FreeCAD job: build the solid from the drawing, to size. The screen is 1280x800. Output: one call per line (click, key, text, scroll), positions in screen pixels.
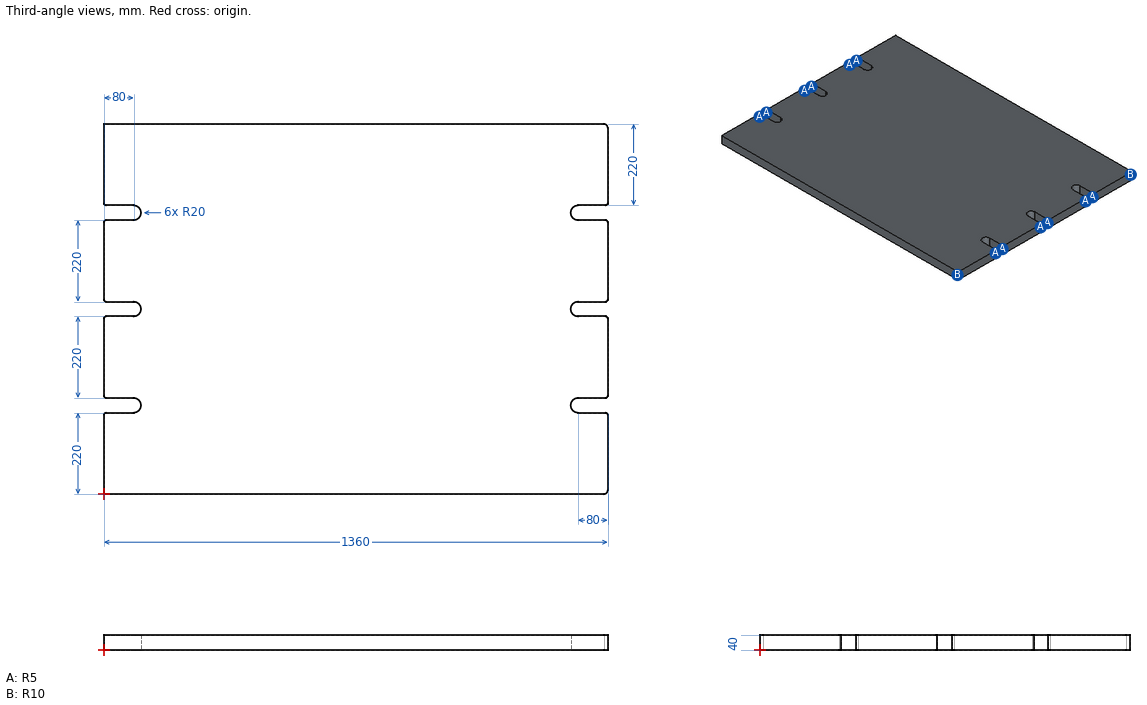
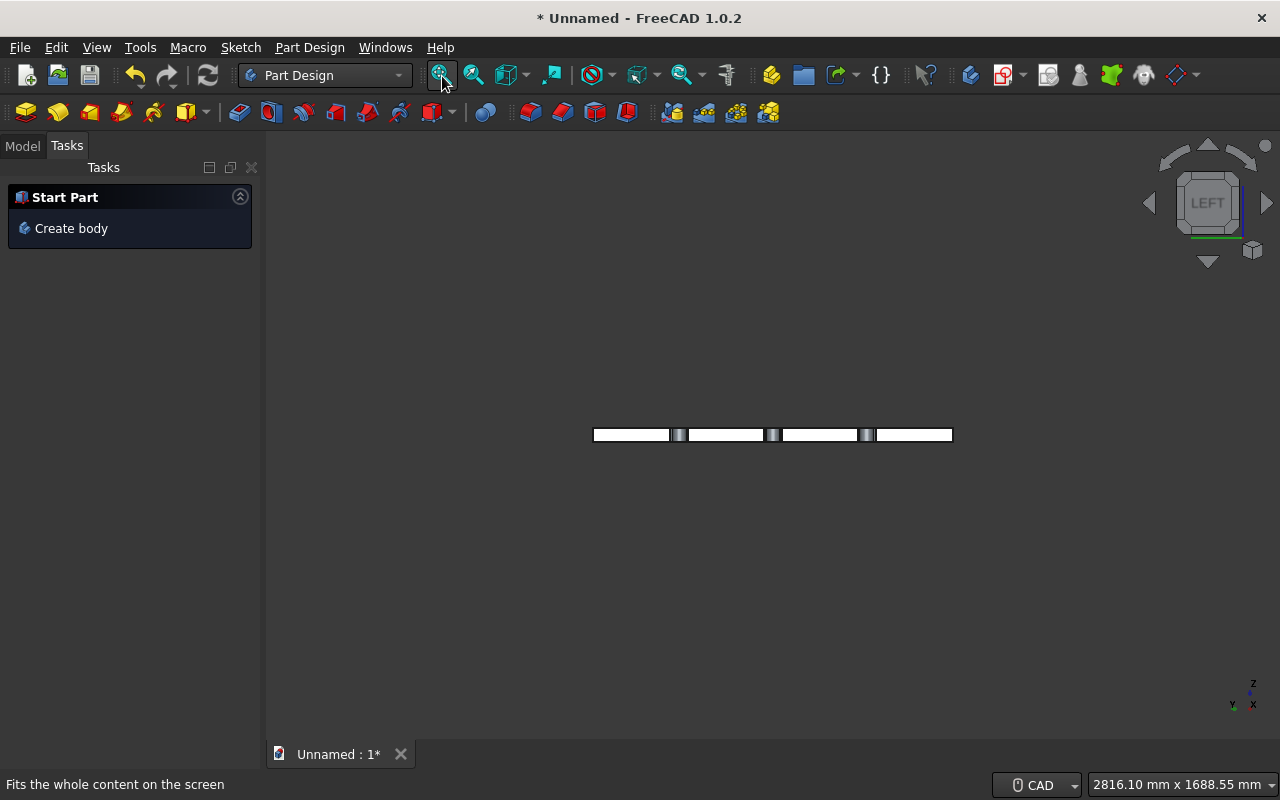
scroll(593, 434, up, 6)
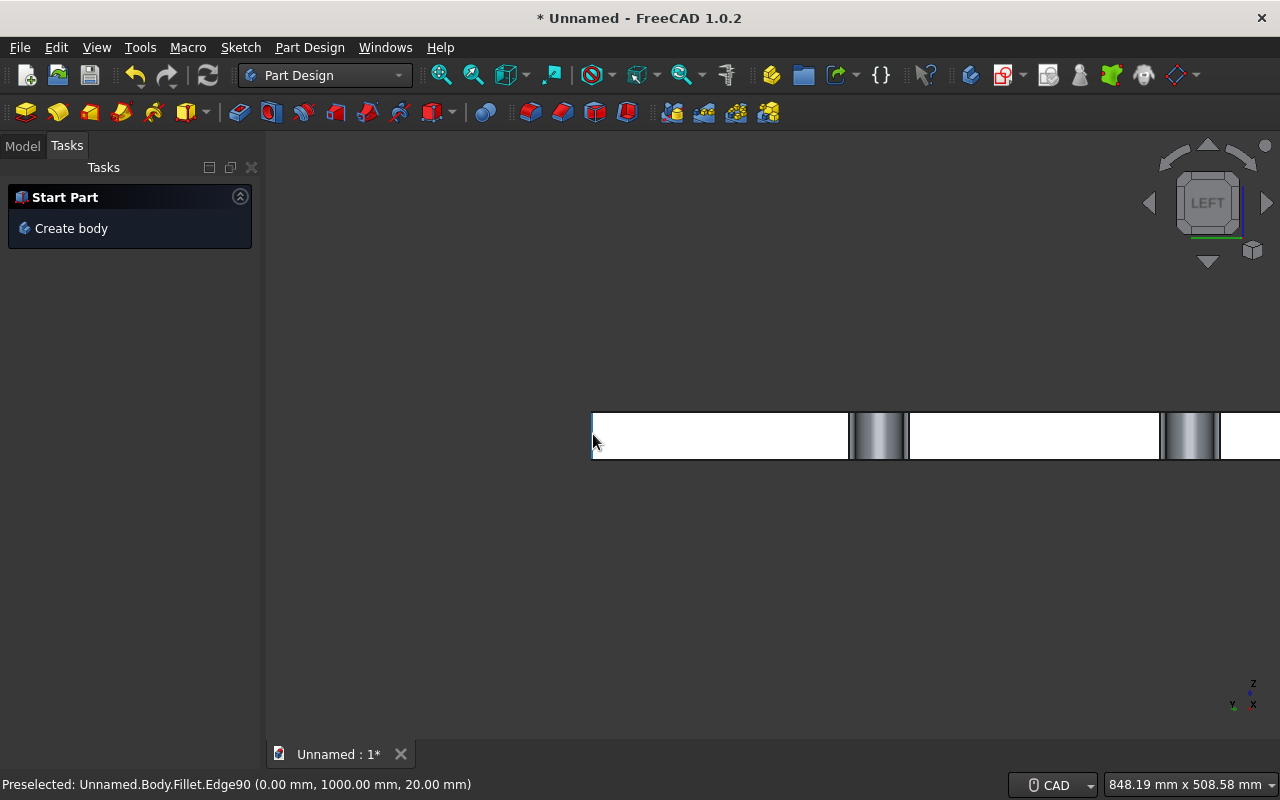
click(442, 76)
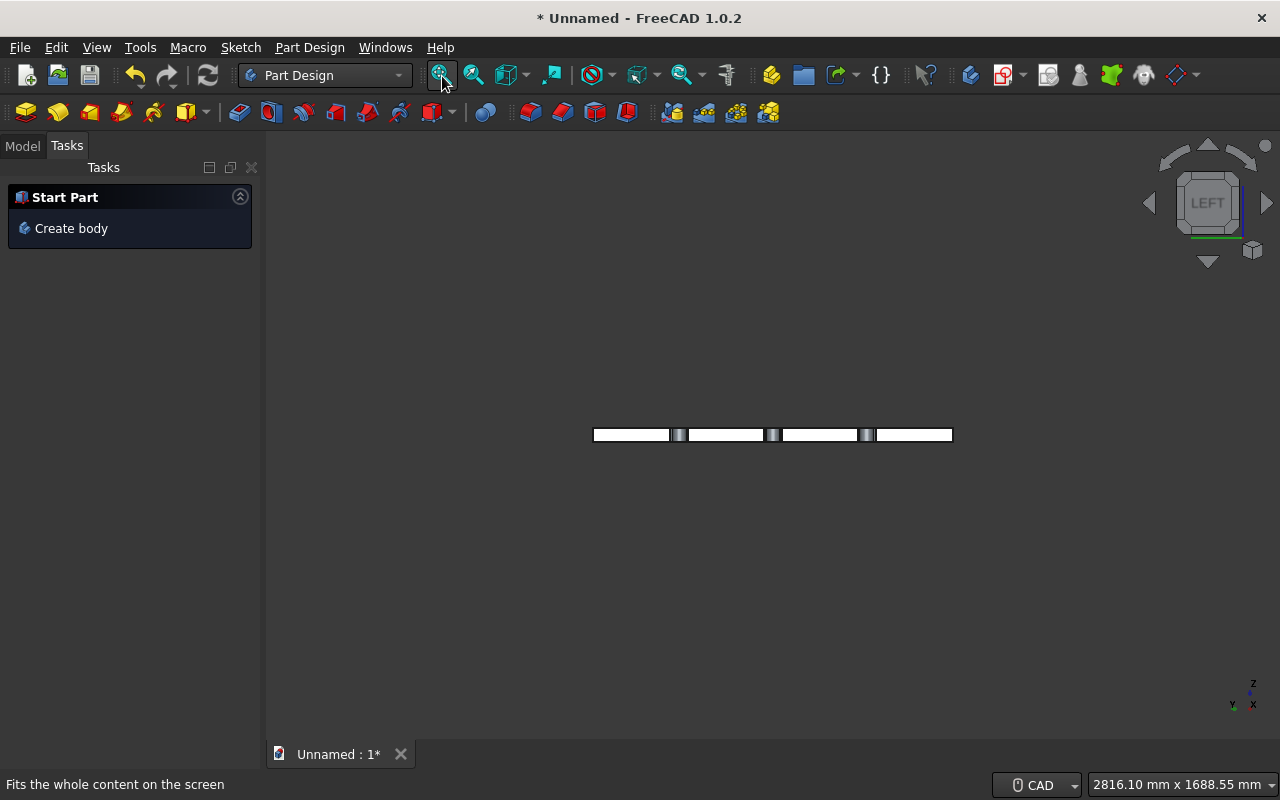
key(0)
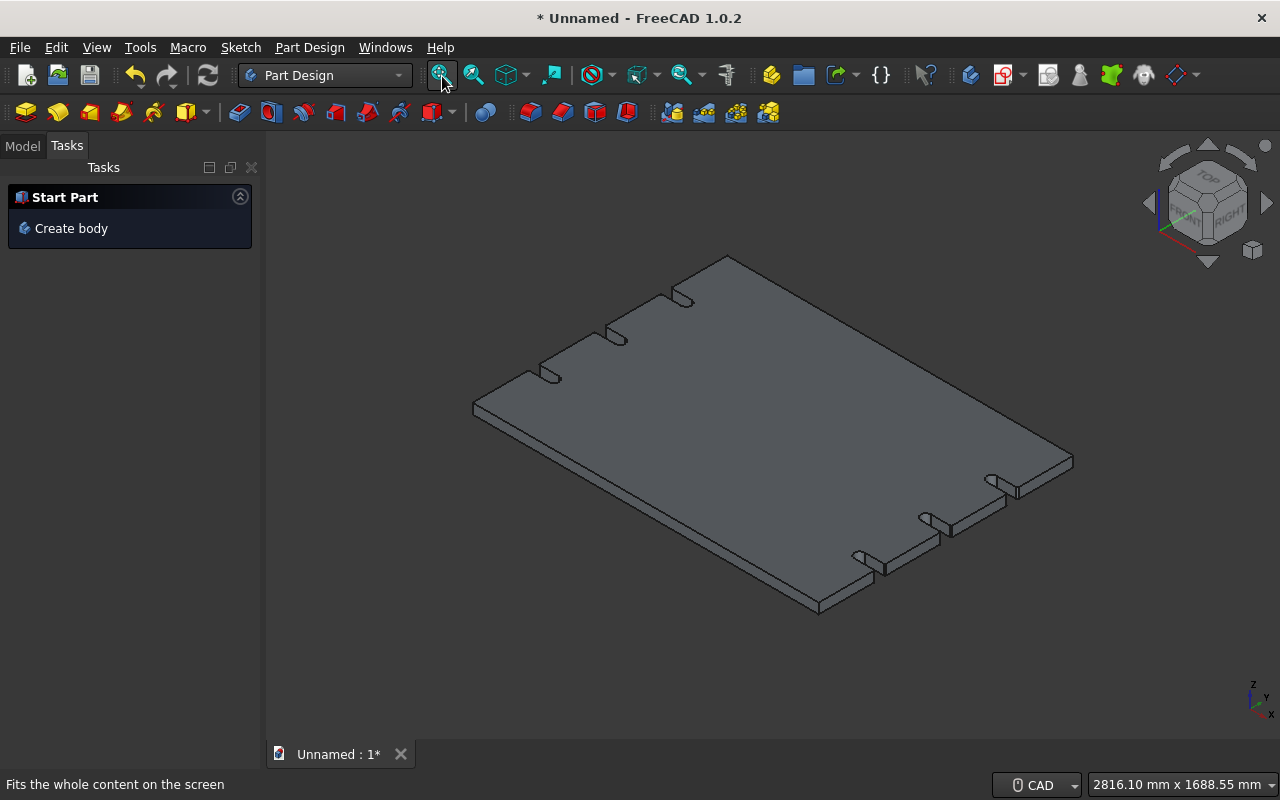
click(819, 609)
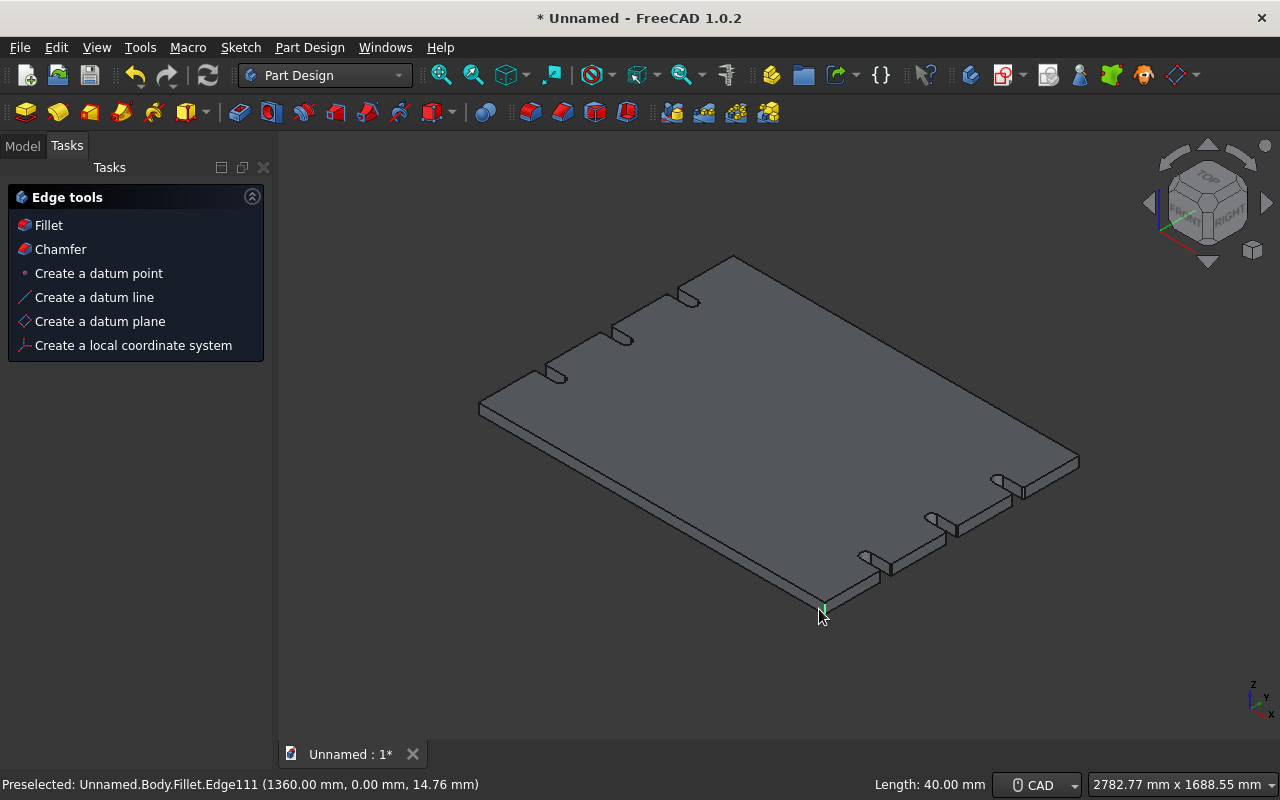
scroll(1079, 460, up, 6)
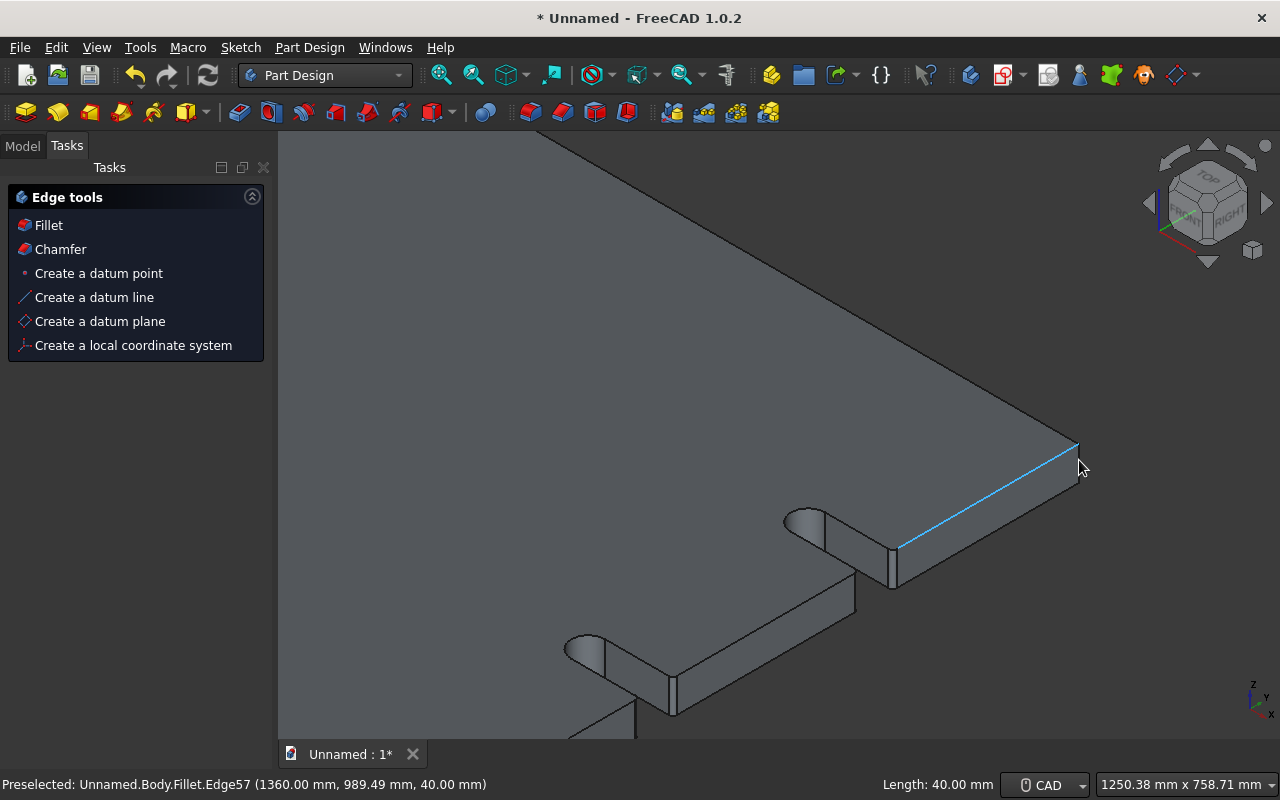
click(442, 76)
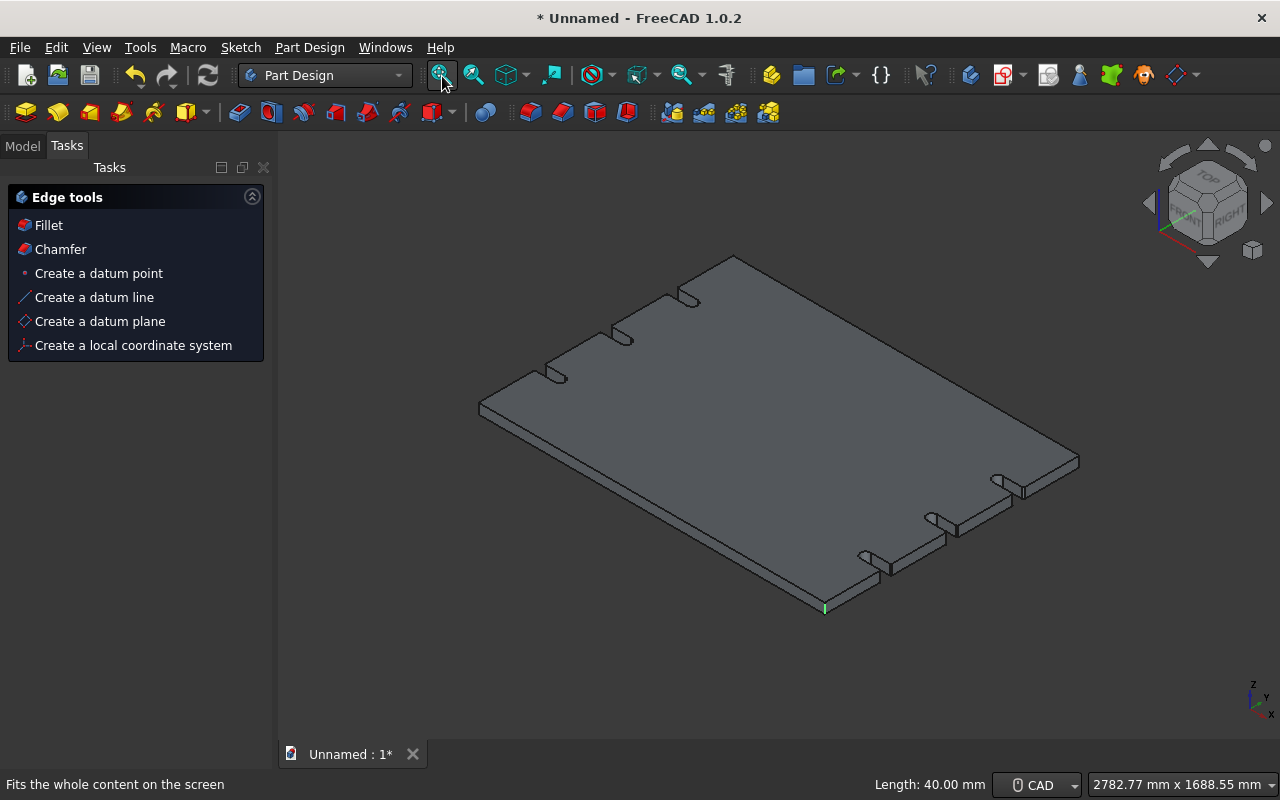
key(2)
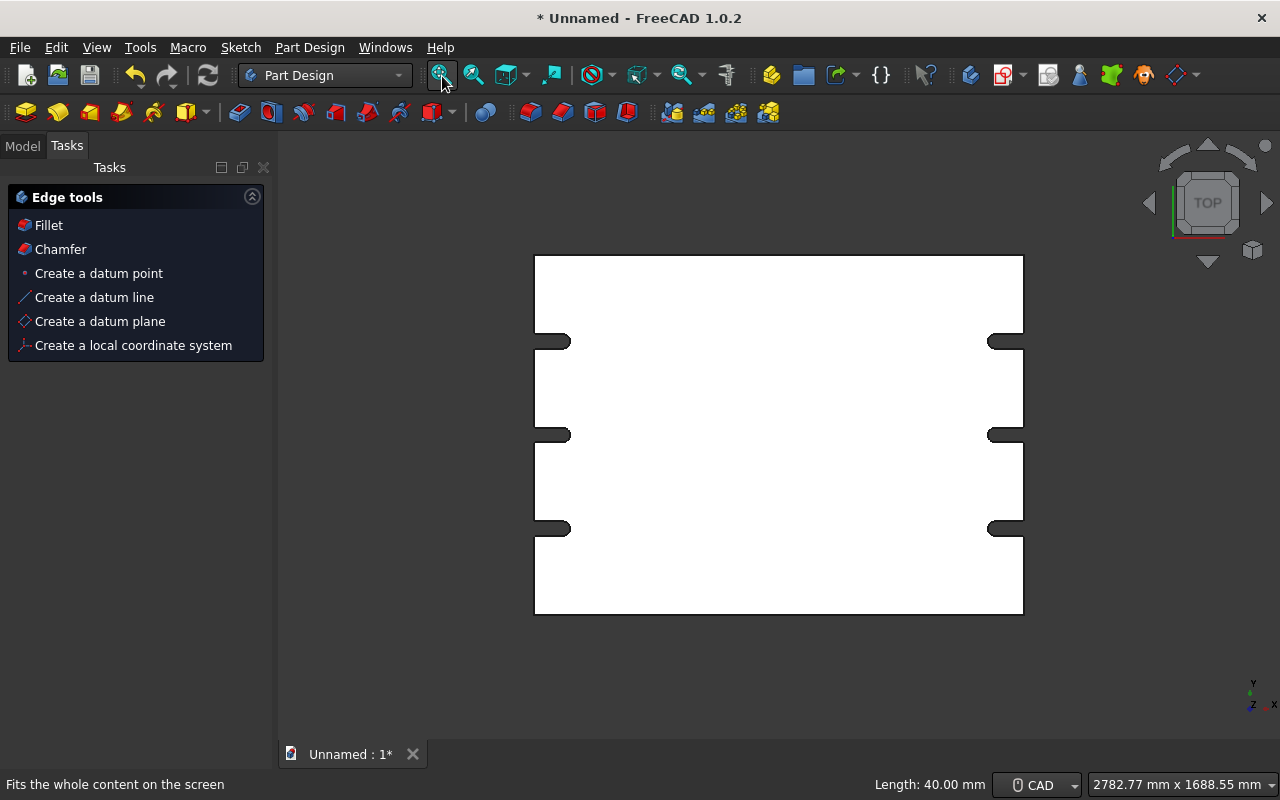
scroll(1024, 254, up, 6)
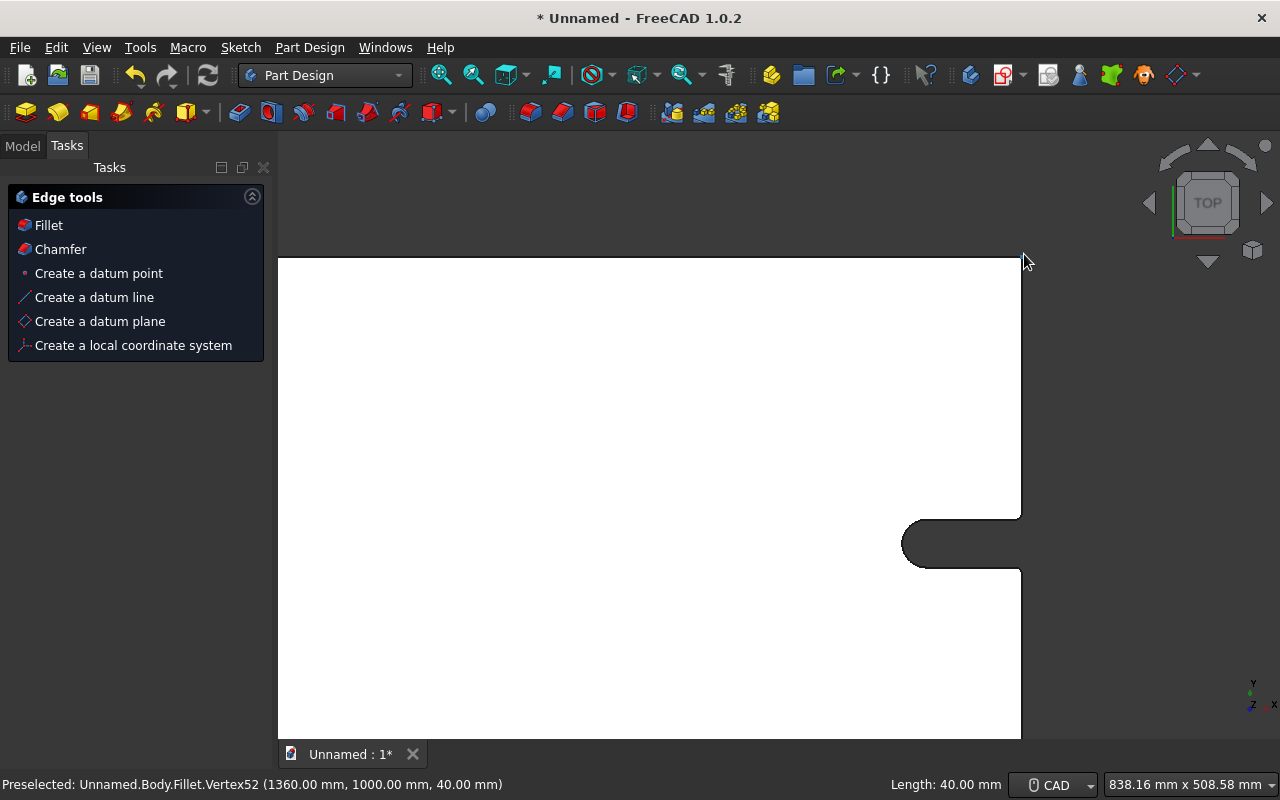
click(442, 76)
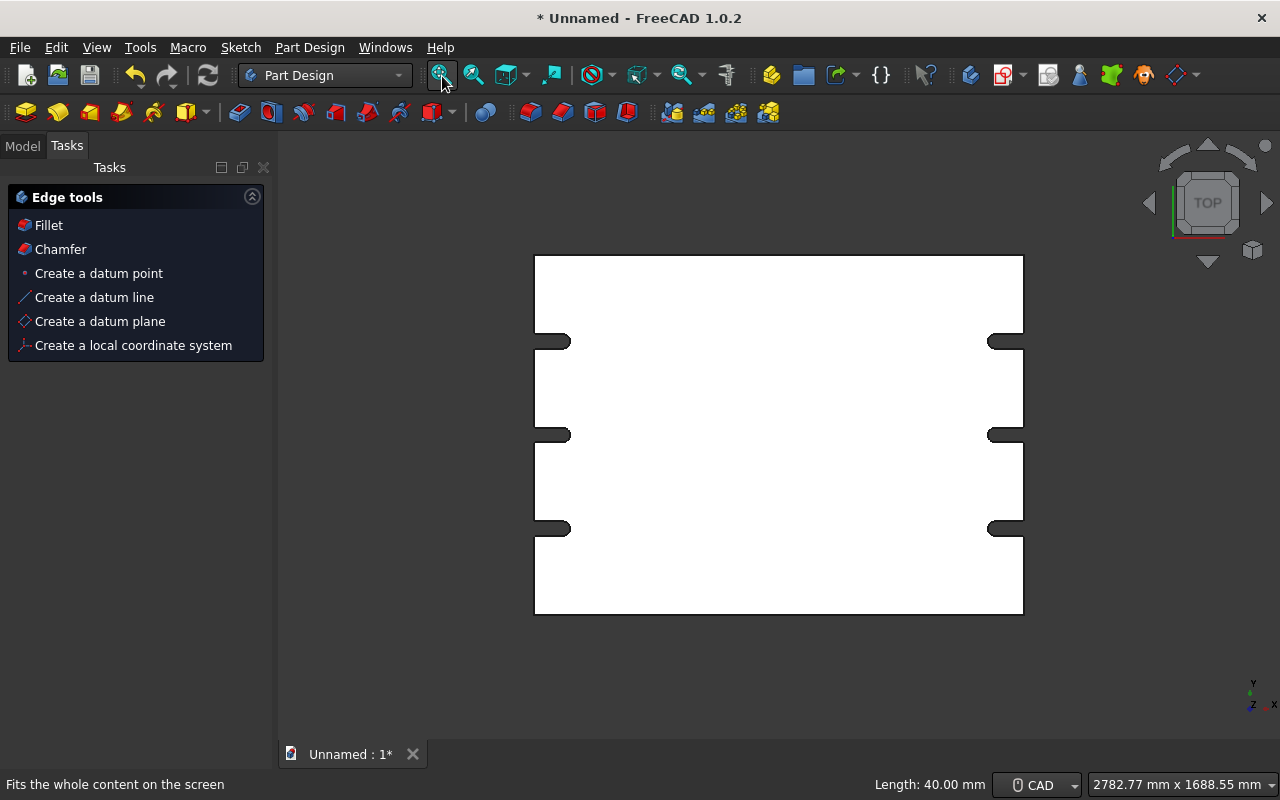
key(1)